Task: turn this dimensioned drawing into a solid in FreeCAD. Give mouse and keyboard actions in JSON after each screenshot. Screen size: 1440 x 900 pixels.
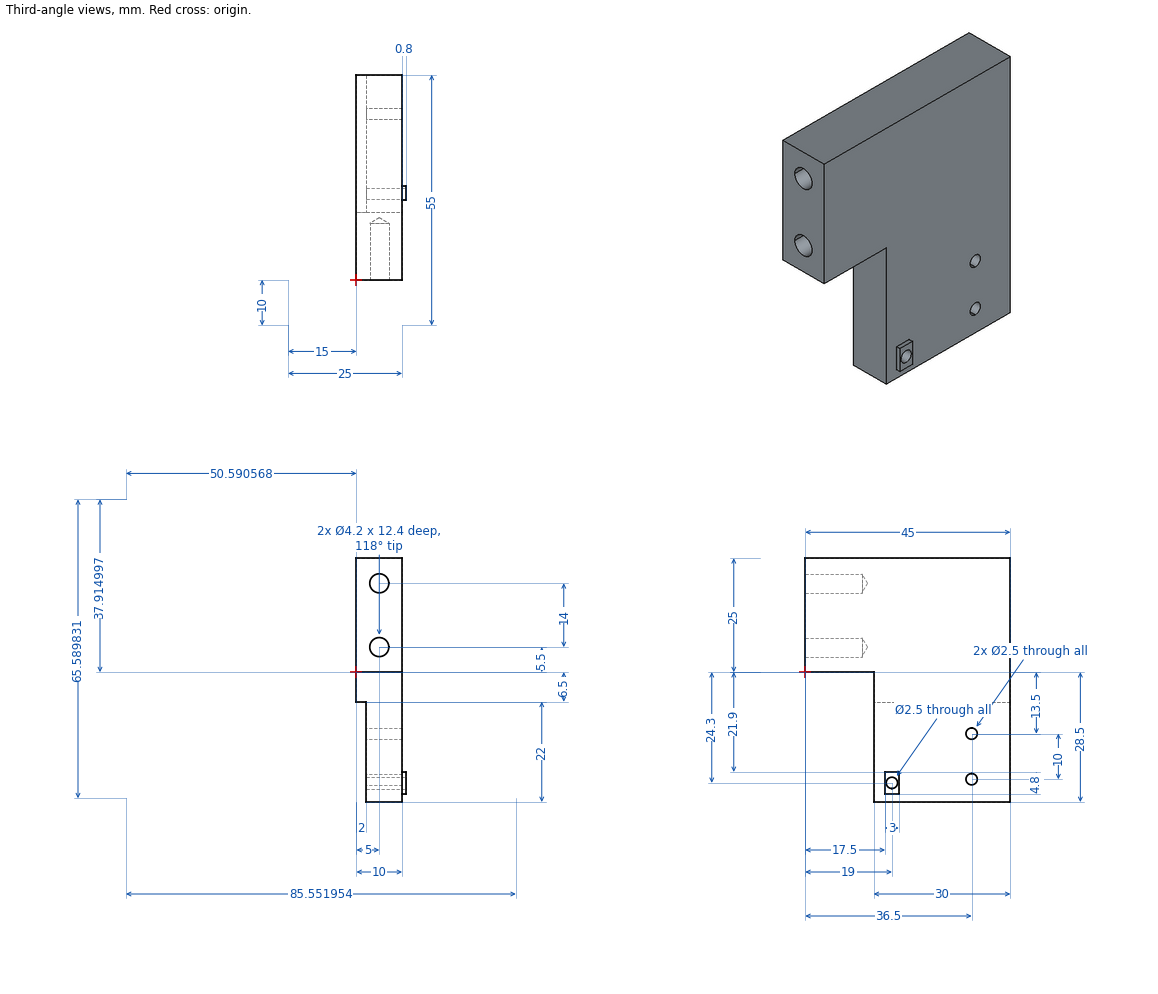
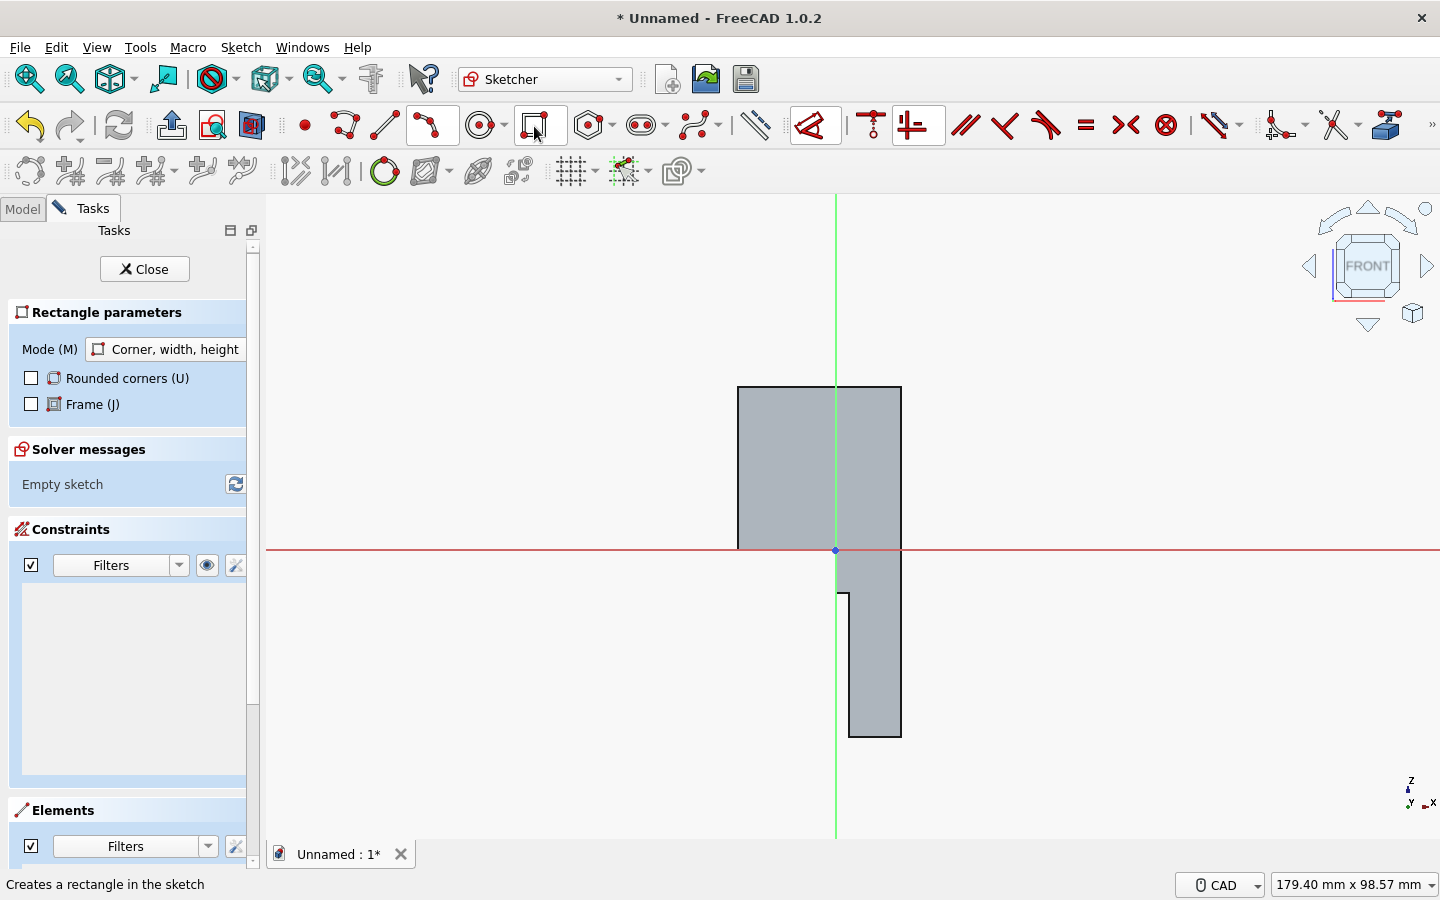
{"action": "left_click", "coordinate": [505, 302]}
{"action": "left_click", "coordinate": [1064, 731]}
{"action": "key", "text": "Escape"}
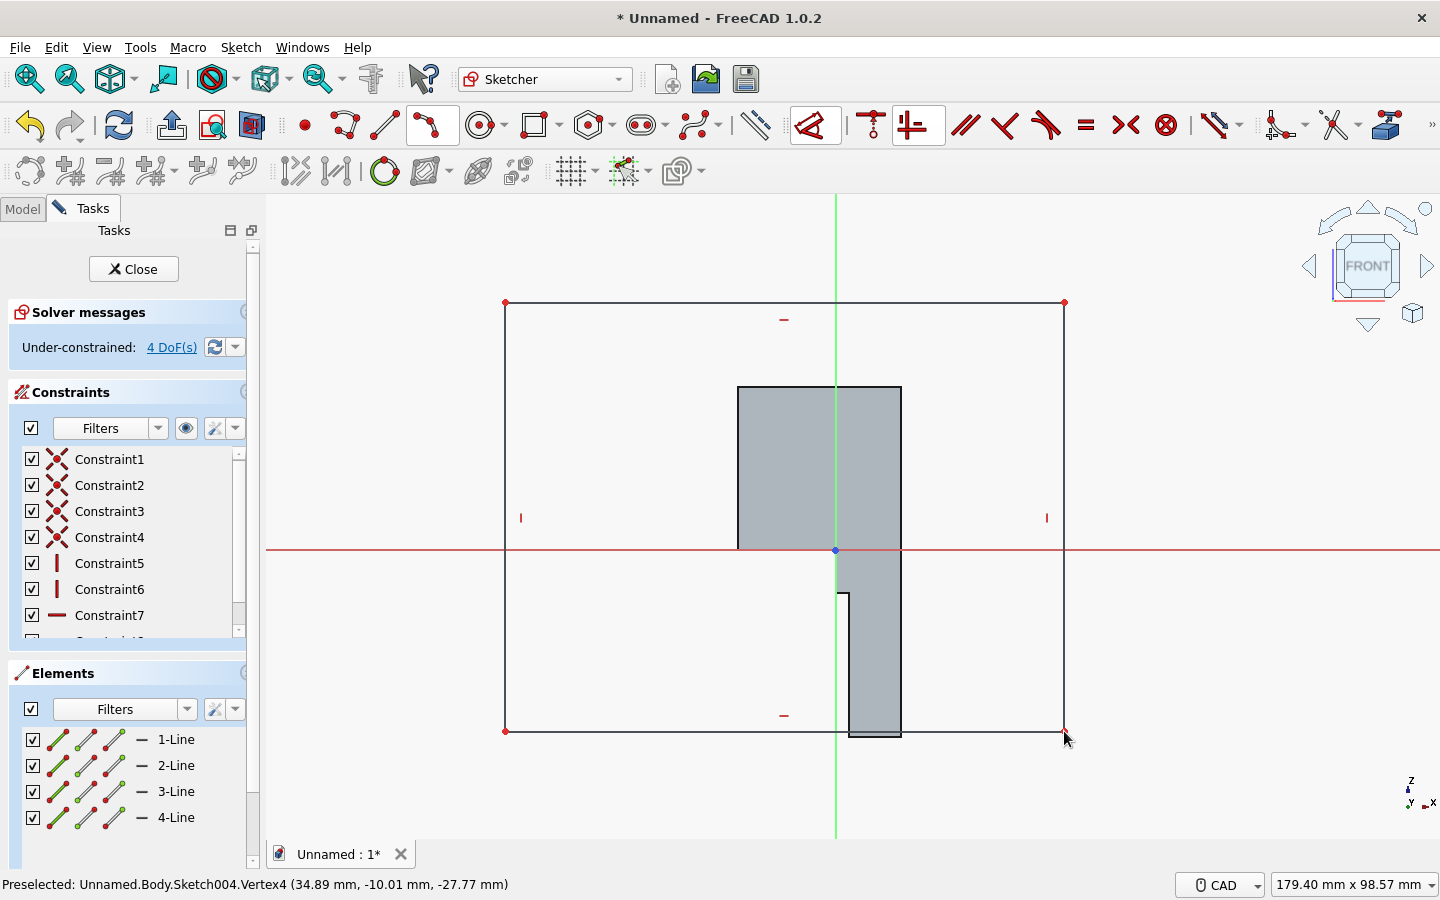
{"action": "left_click", "coordinate": [505, 432]}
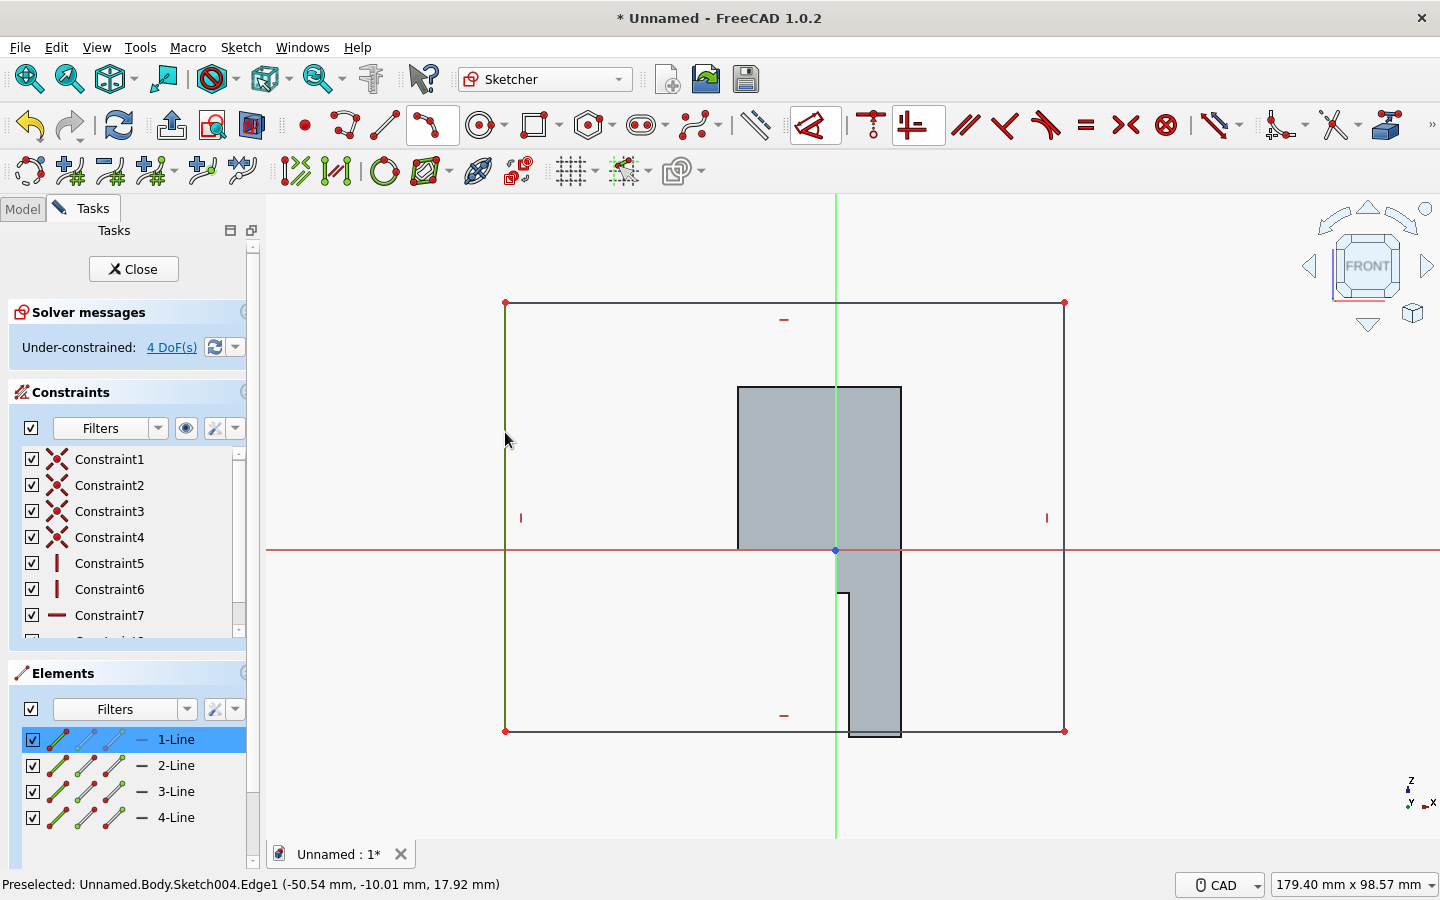
{"action": "key", "text": "i"}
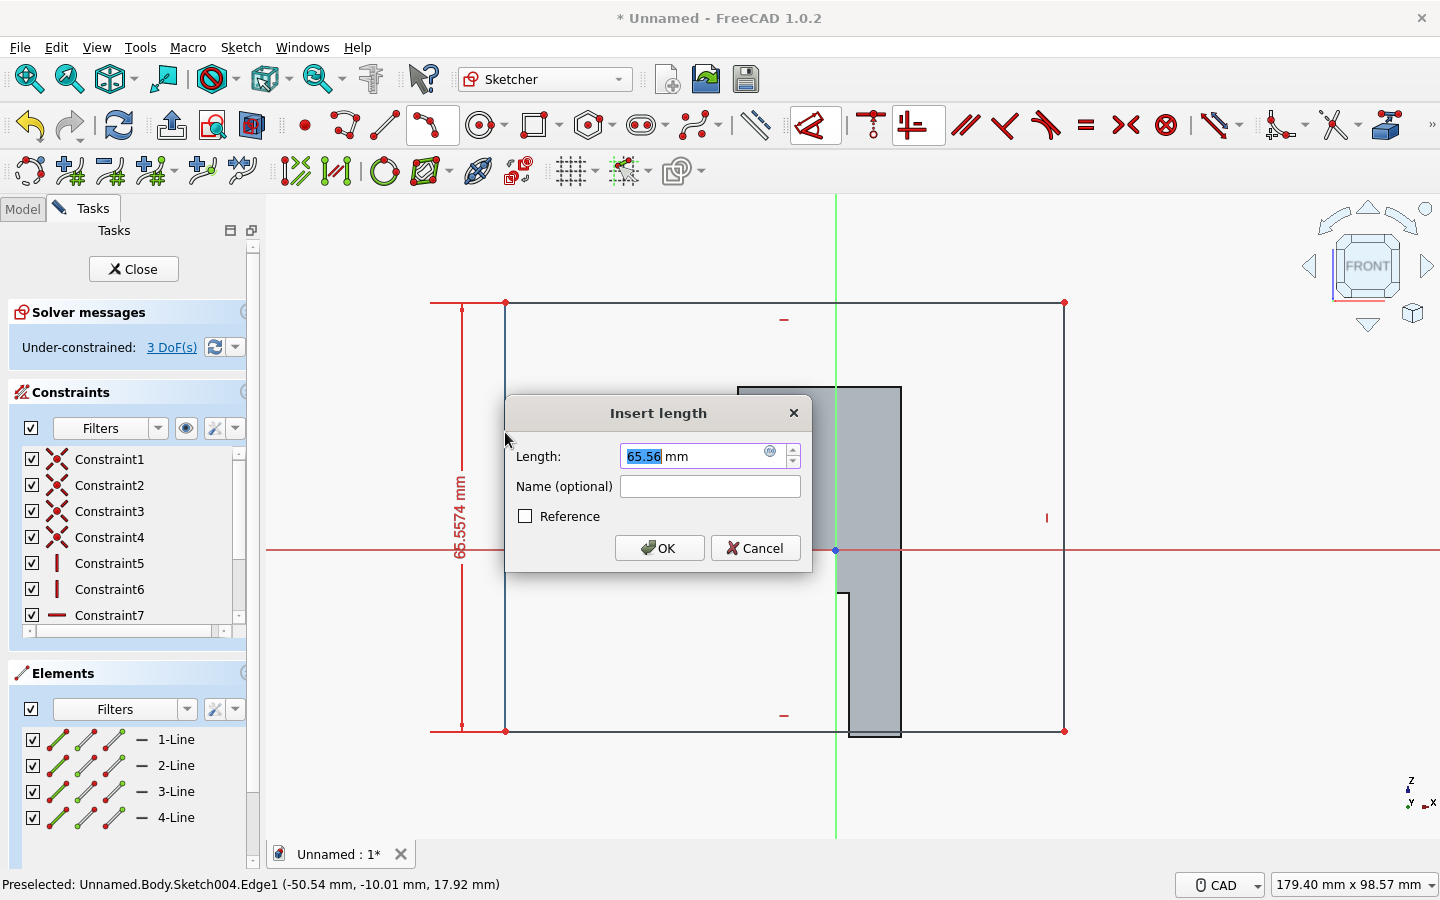
{"action": "type", "text": "65.589831"}
{"action": "key", "text": "Return"}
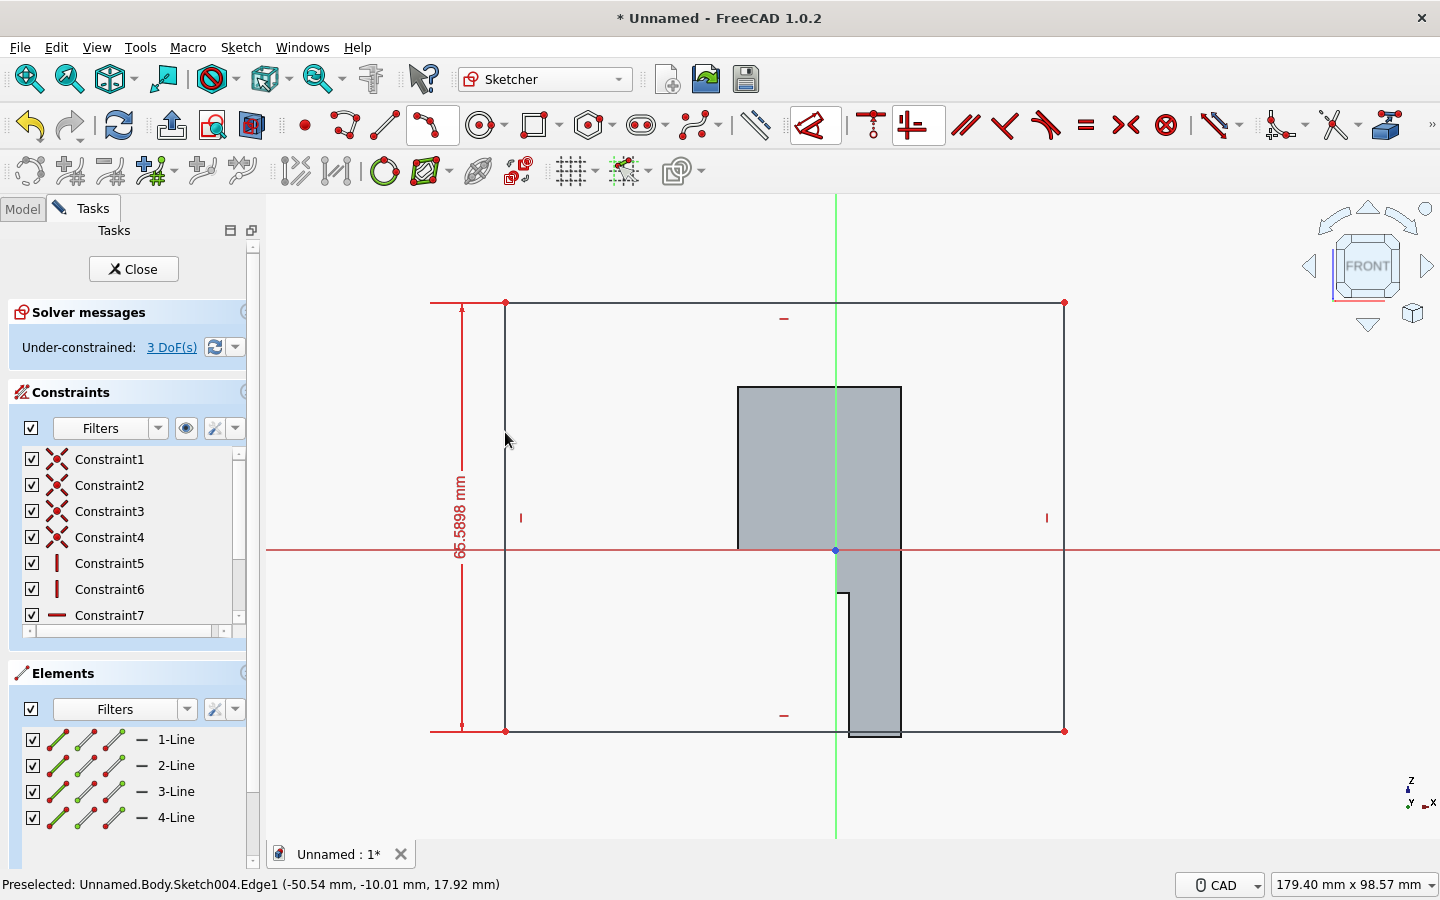
{"action": "left_click", "coordinate": [673, 732]}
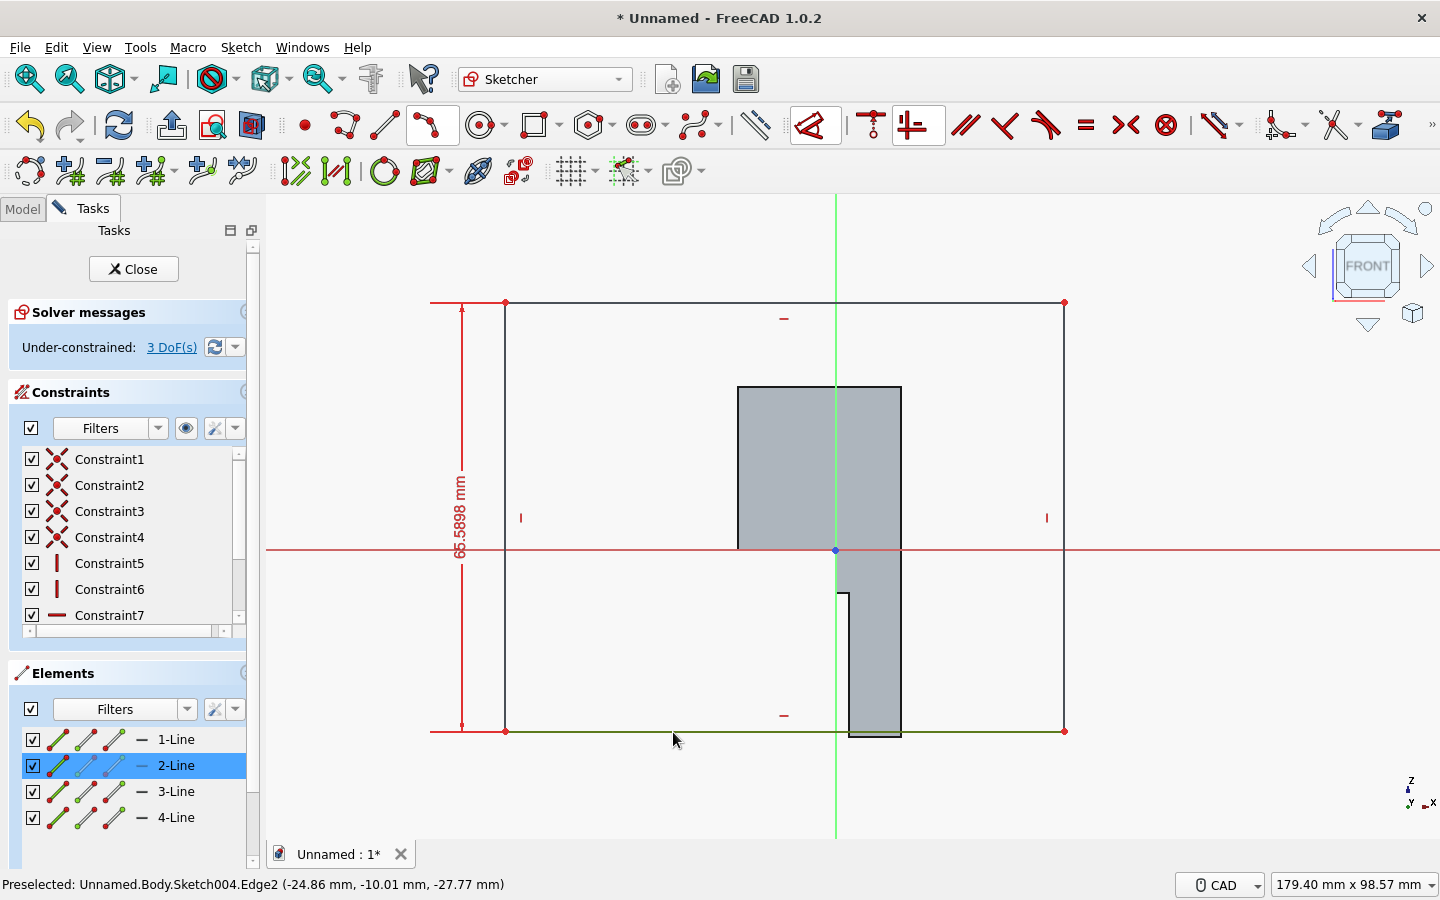
{"action": "left_click", "coordinate": [836, 126]}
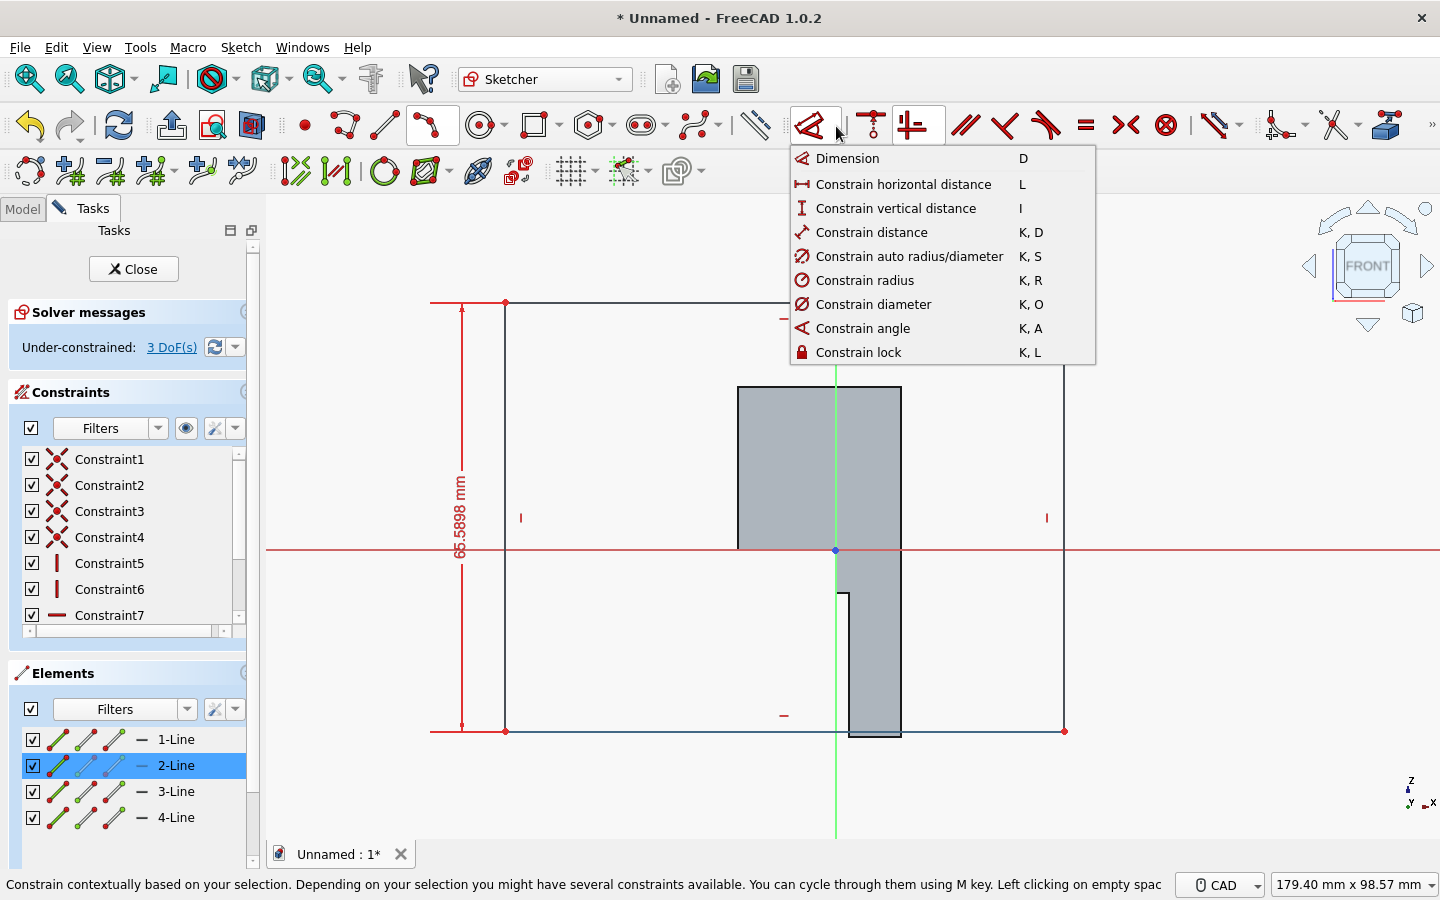
{"action": "left_click", "coordinate": [943, 184]}